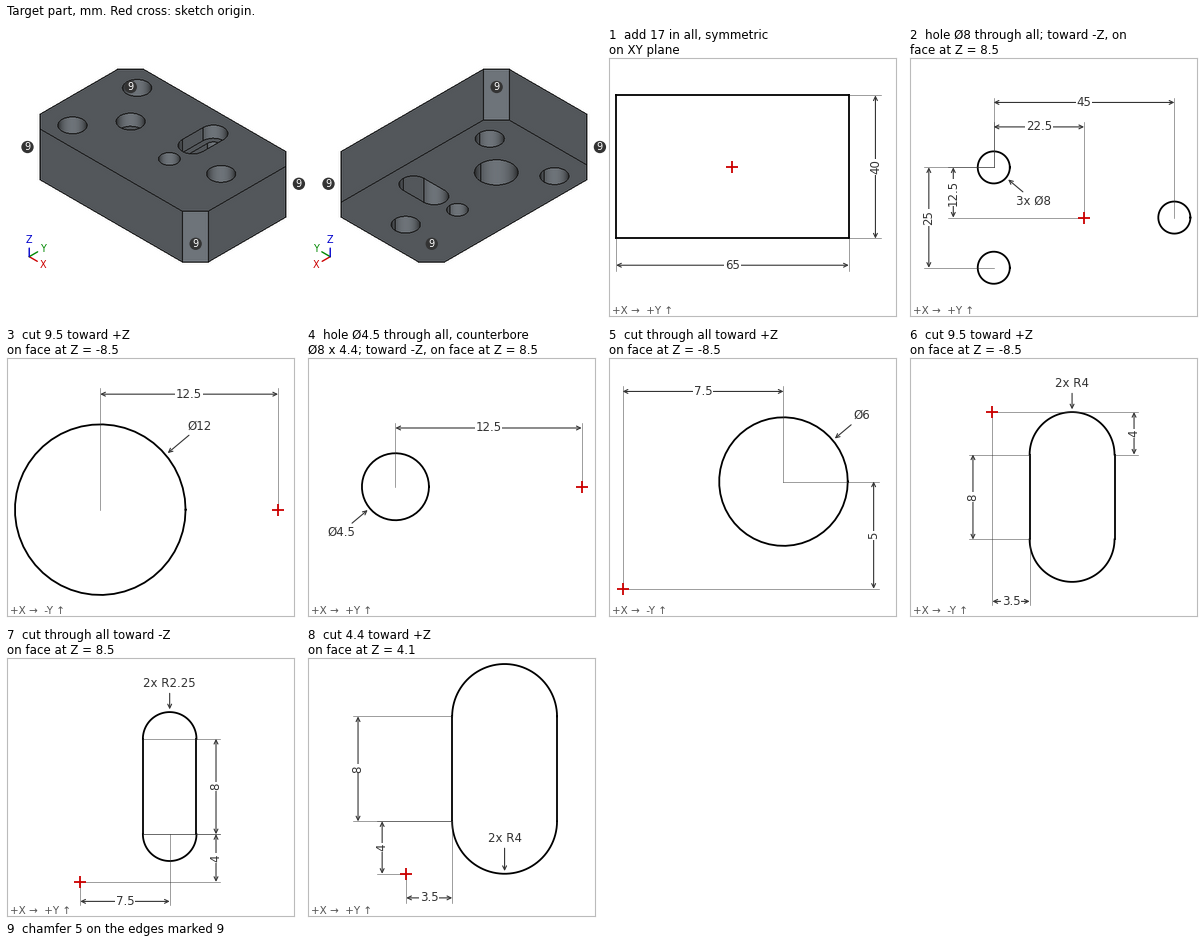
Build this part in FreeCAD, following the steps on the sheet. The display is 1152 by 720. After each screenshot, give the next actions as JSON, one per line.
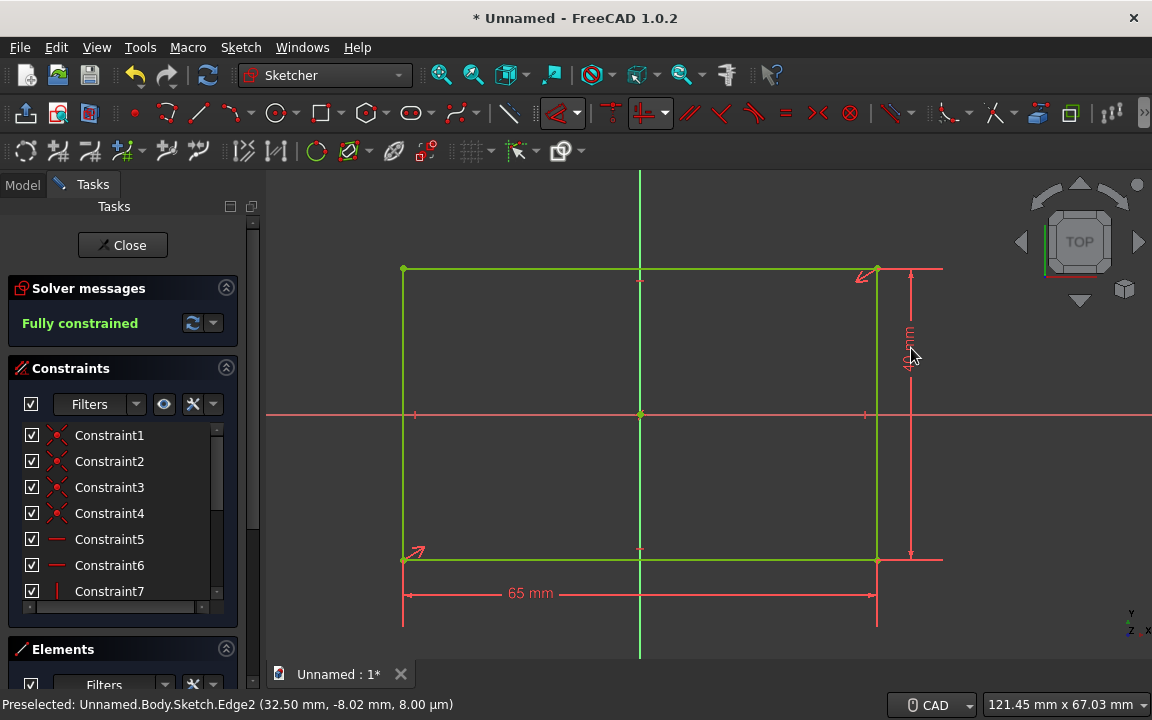
{"action": "left_click", "coordinate": [123, 245]}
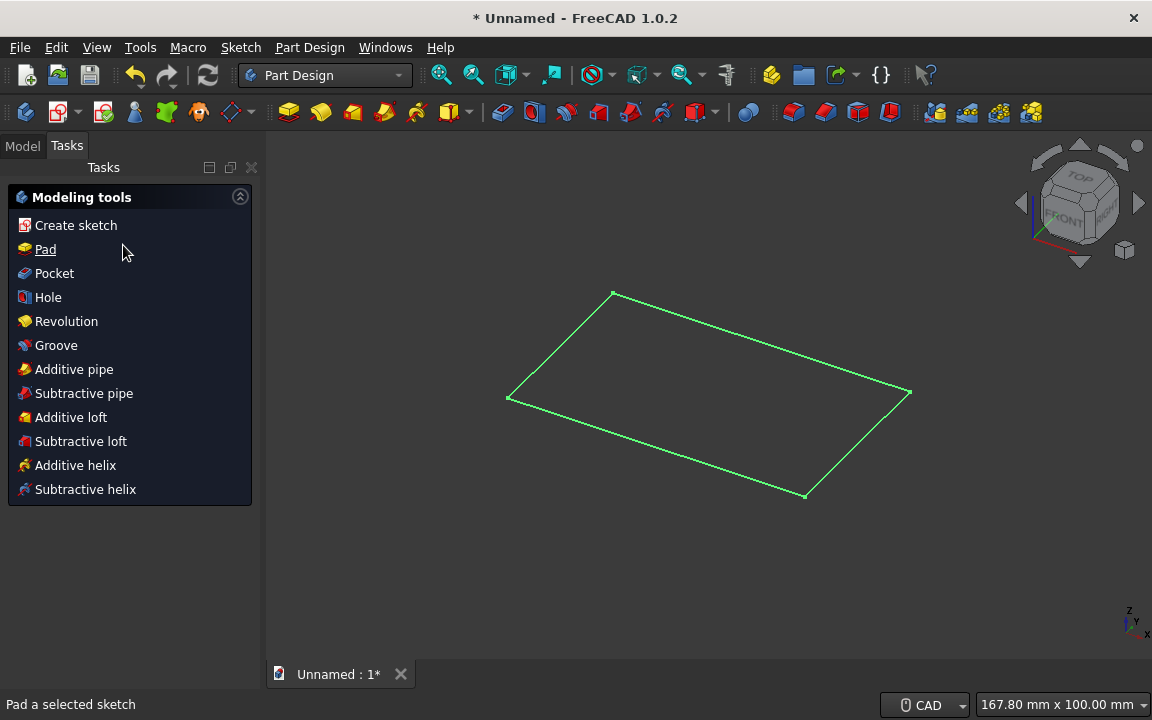
{"action": "left_click", "coordinate": [290, 112]}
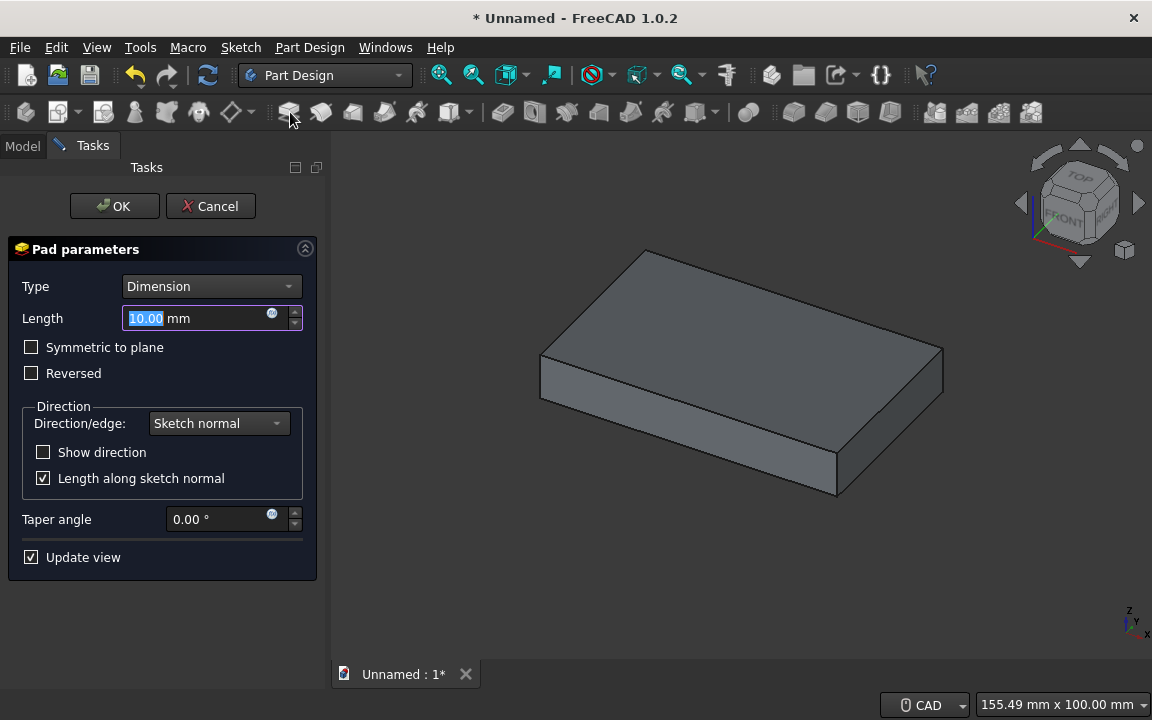
{"action": "type", "text": "17"}
{"action": "key", "text": "Tab"}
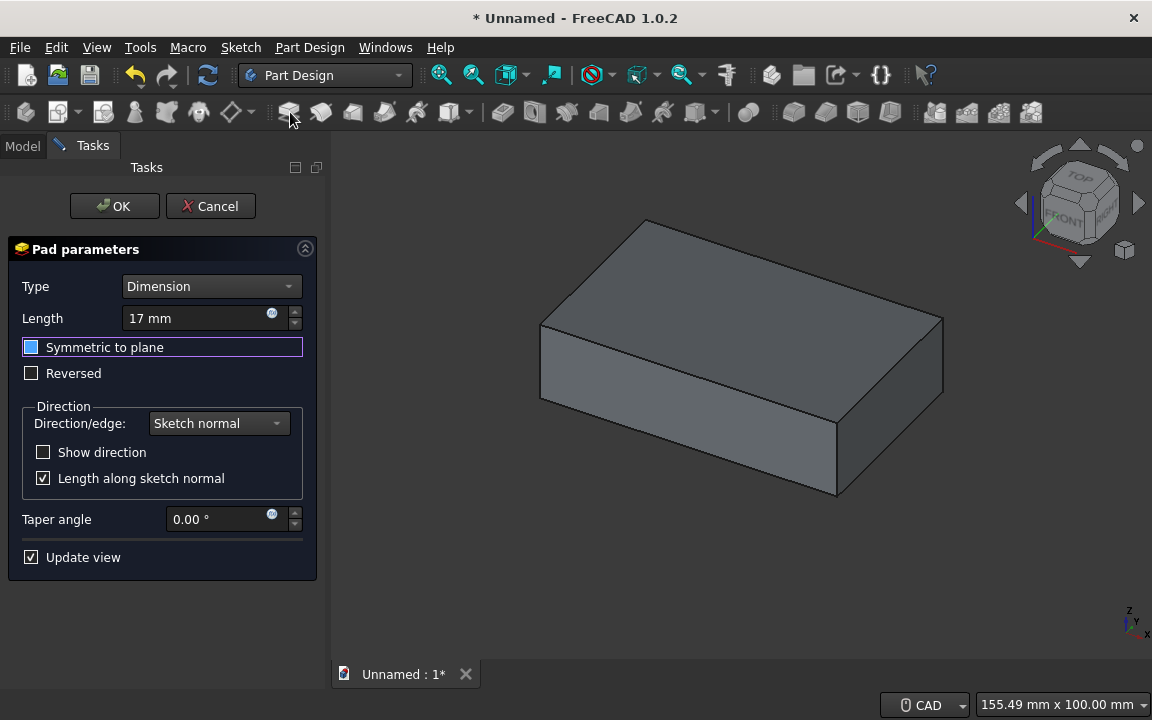
{"action": "left_click", "coordinate": [30, 347]}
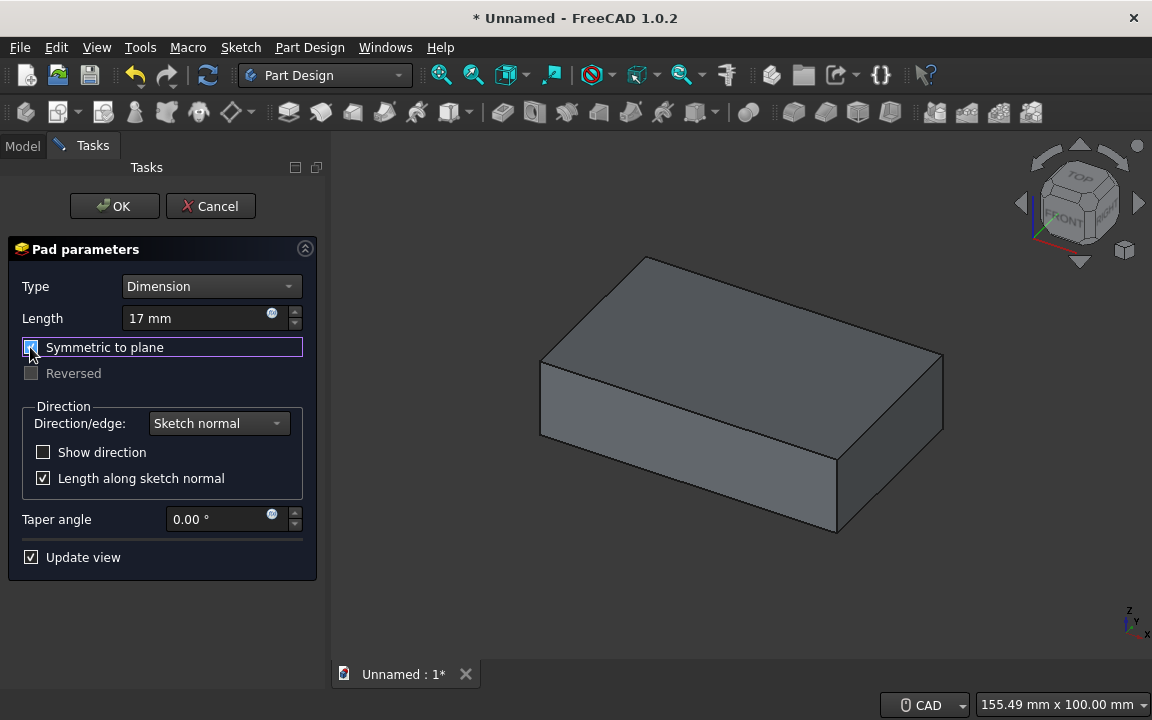
{"action": "left_click", "coordinate": [115, 206]}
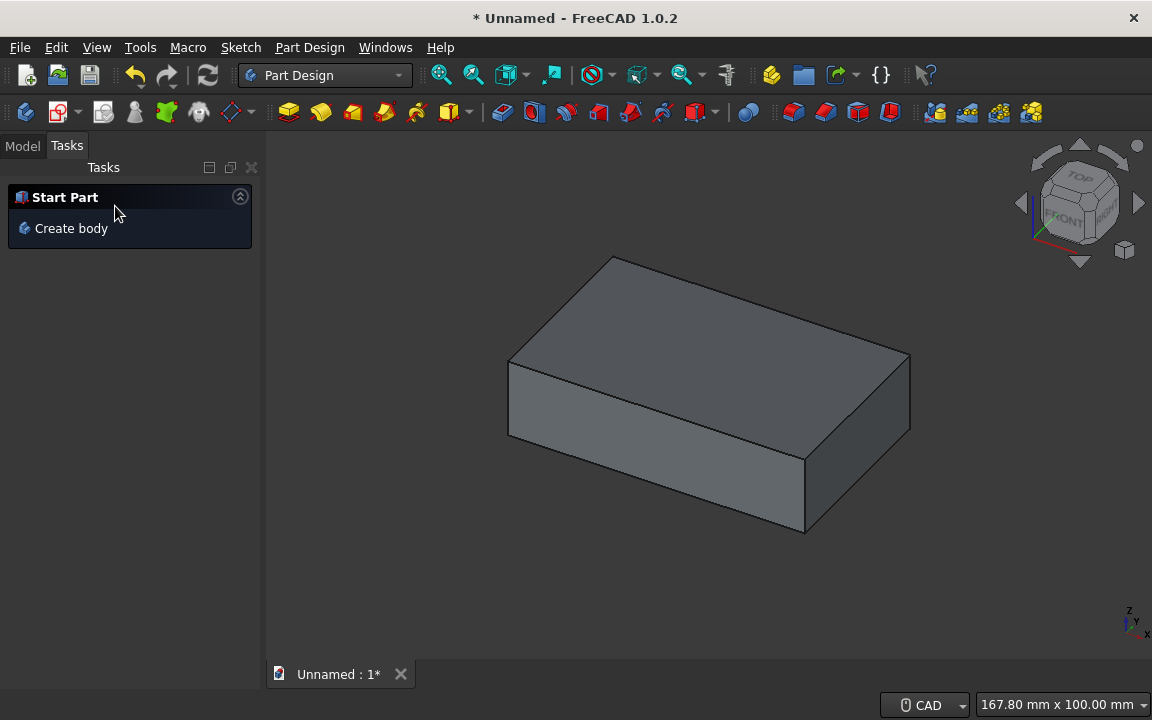
{"action": "left_click", "coordinate": [751, 371]}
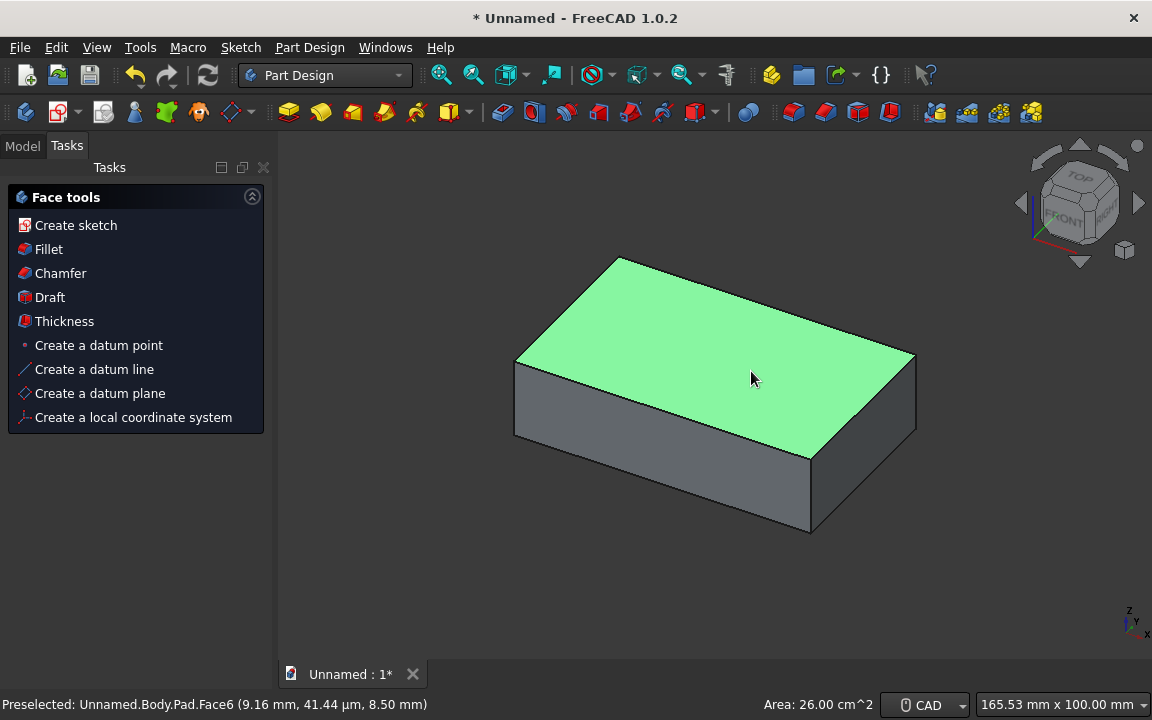
{"action": "left_click", "coordinate": [58, 112]}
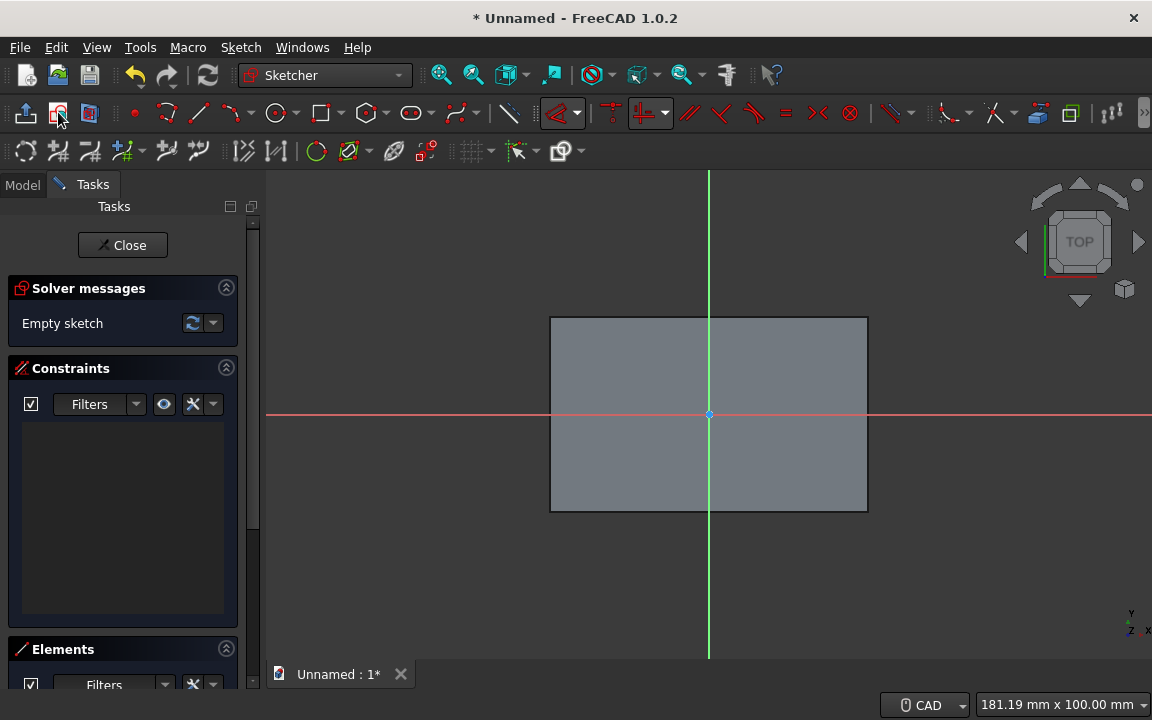
{"action": "scroll", "coordinate": [792, 415], "scroll_direction": "up", "scroll_amount": 3}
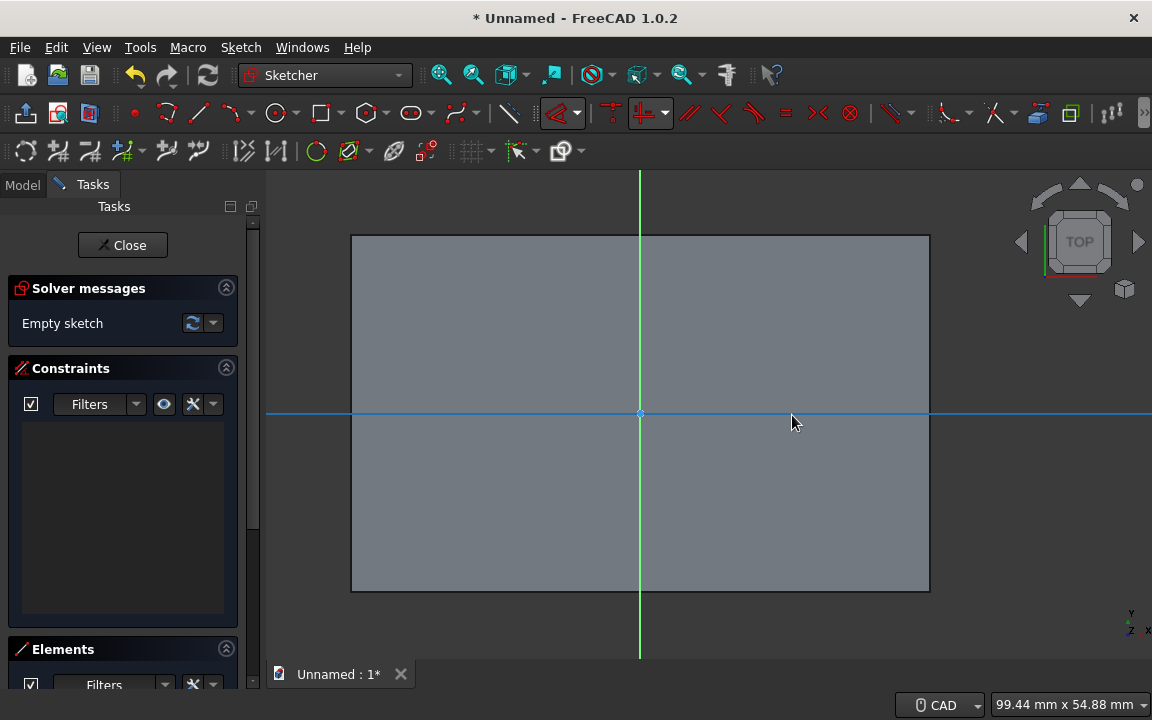
{"action": "left_click", "coordinate": [276, 114]}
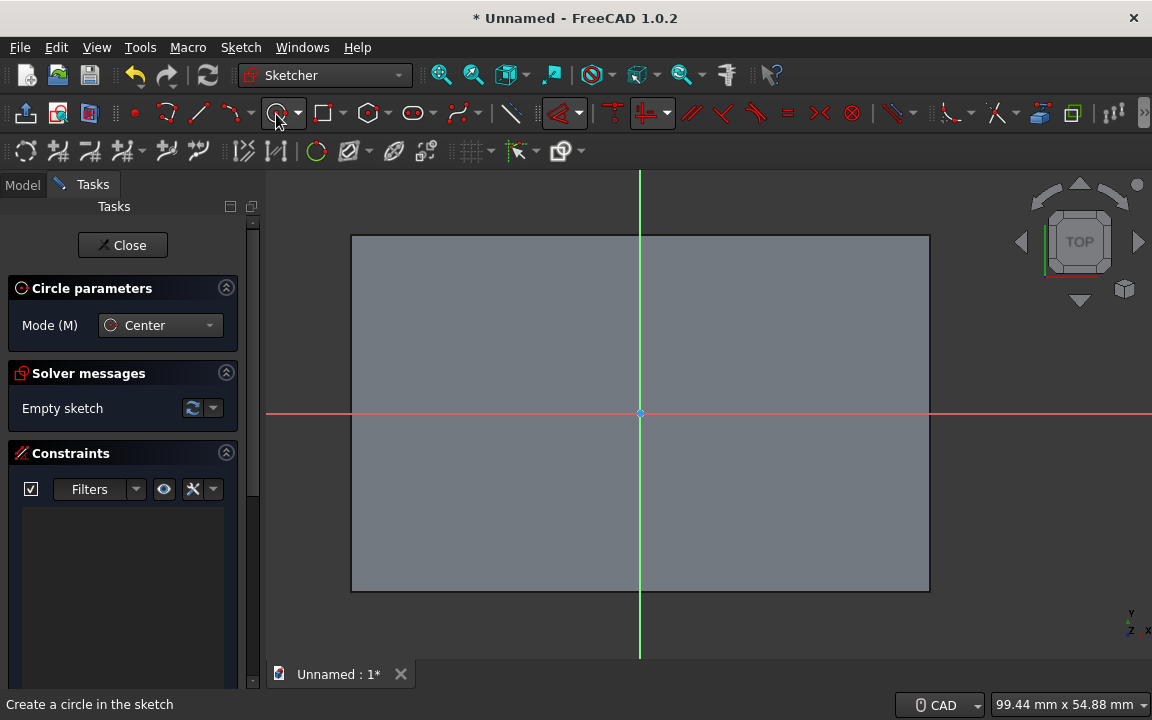
{"action": "left_click", "coordinate": [440, 302]}
{"action": "left_click", "coordinate": [465, 277]}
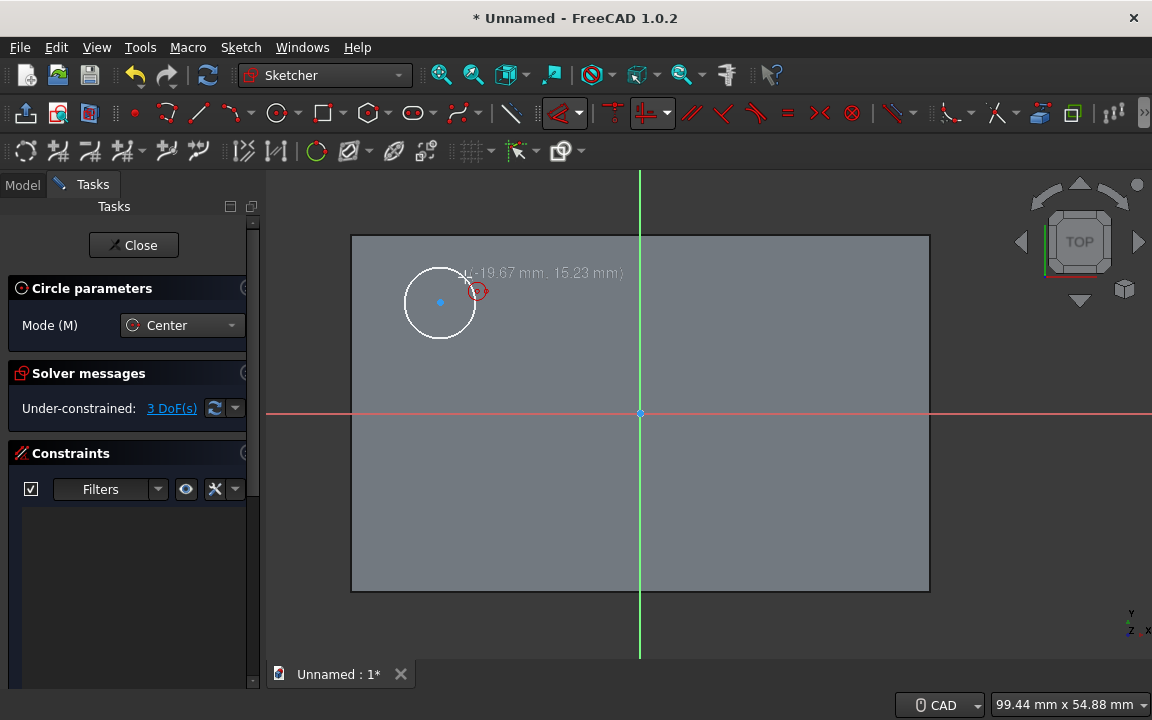
{"action": "left_click", "coordinate": [440, 525]}
{"action": "left_click", "coordinate": [465, 500]}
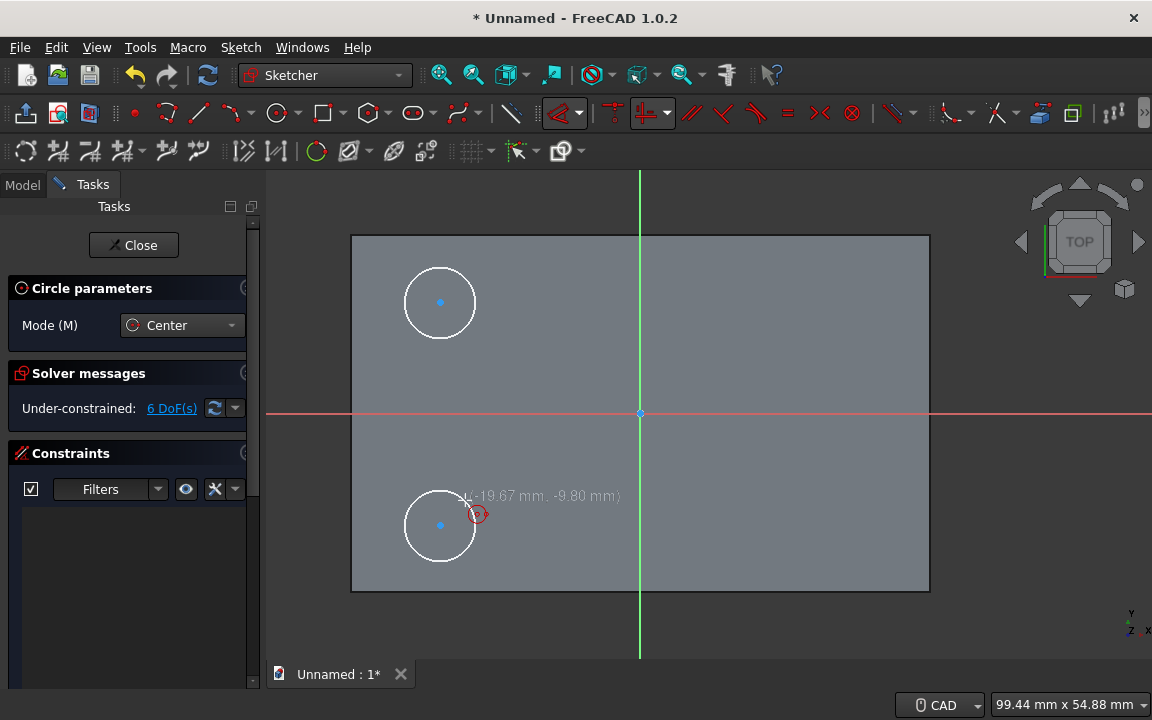
{"action": "left_click", "coordinate": [841, 414]}
{"action": "left_click", "coordinate": [866, 388]}
{"action": "key", "text": "Escape"}